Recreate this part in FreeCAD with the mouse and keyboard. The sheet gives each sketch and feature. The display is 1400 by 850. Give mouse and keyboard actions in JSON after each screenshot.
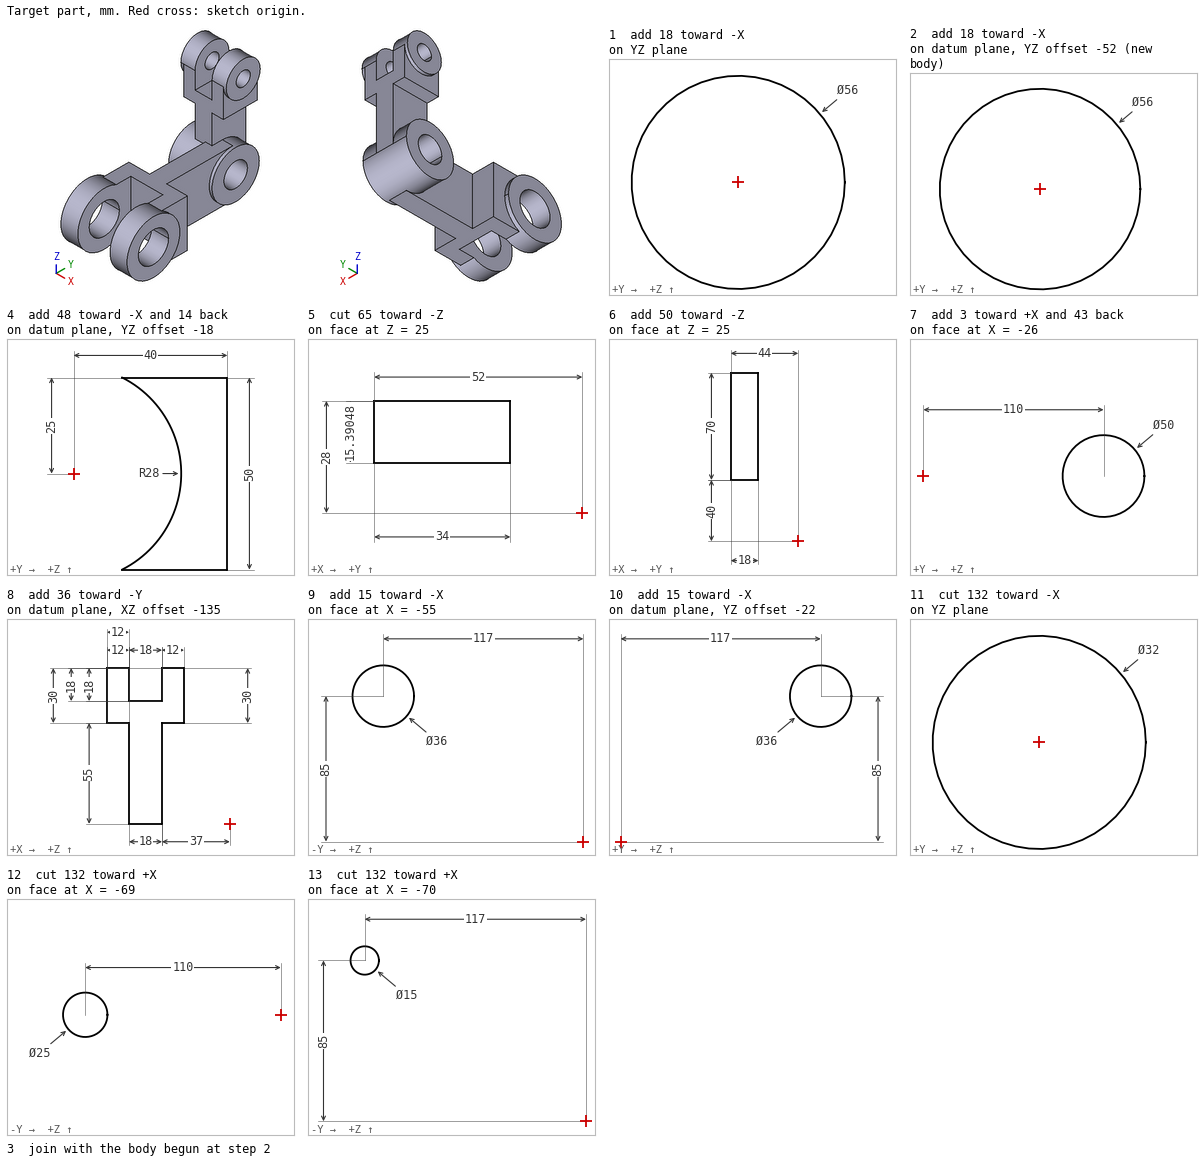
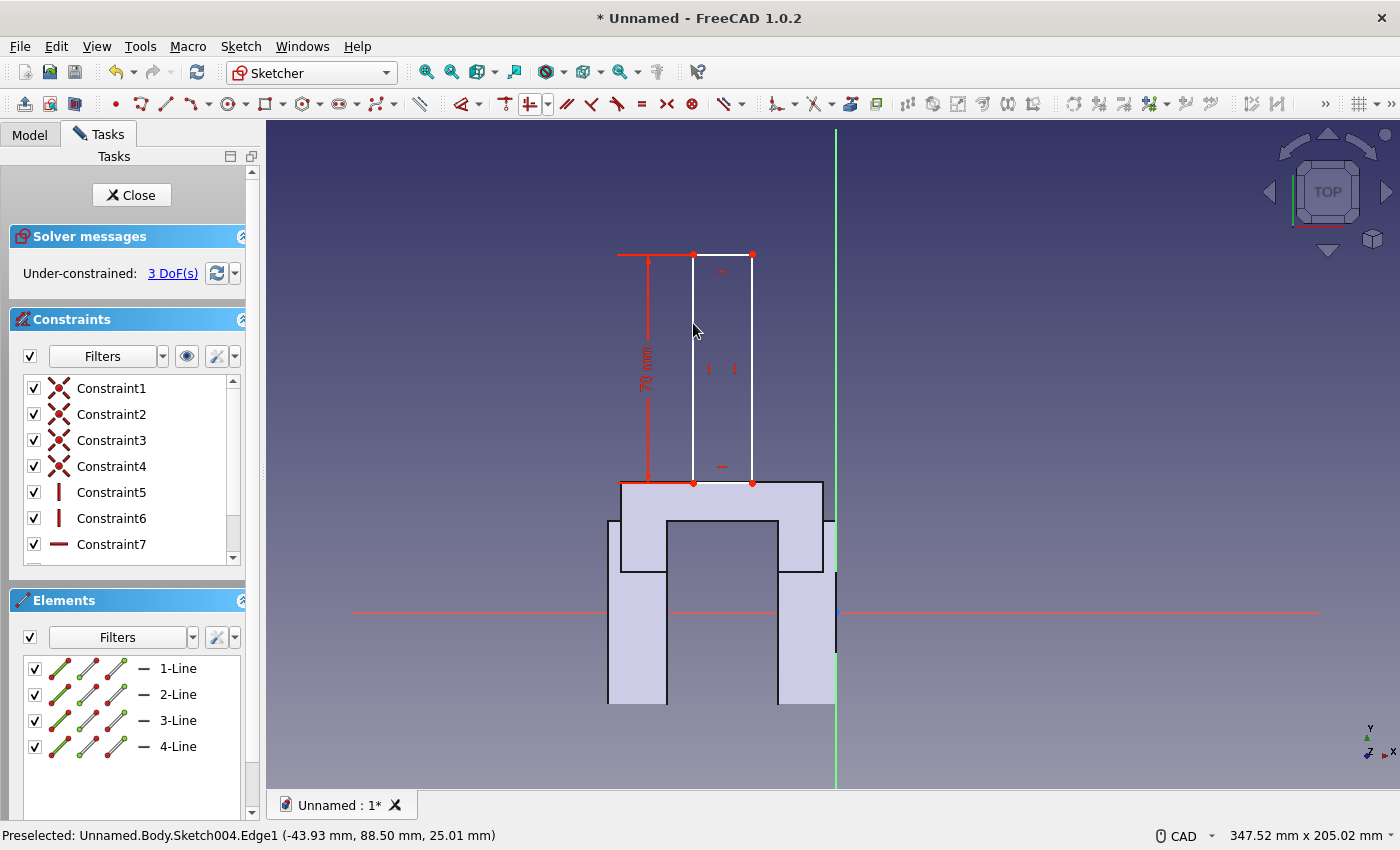
{"action": "left_click", "coordinate": [711, 483]}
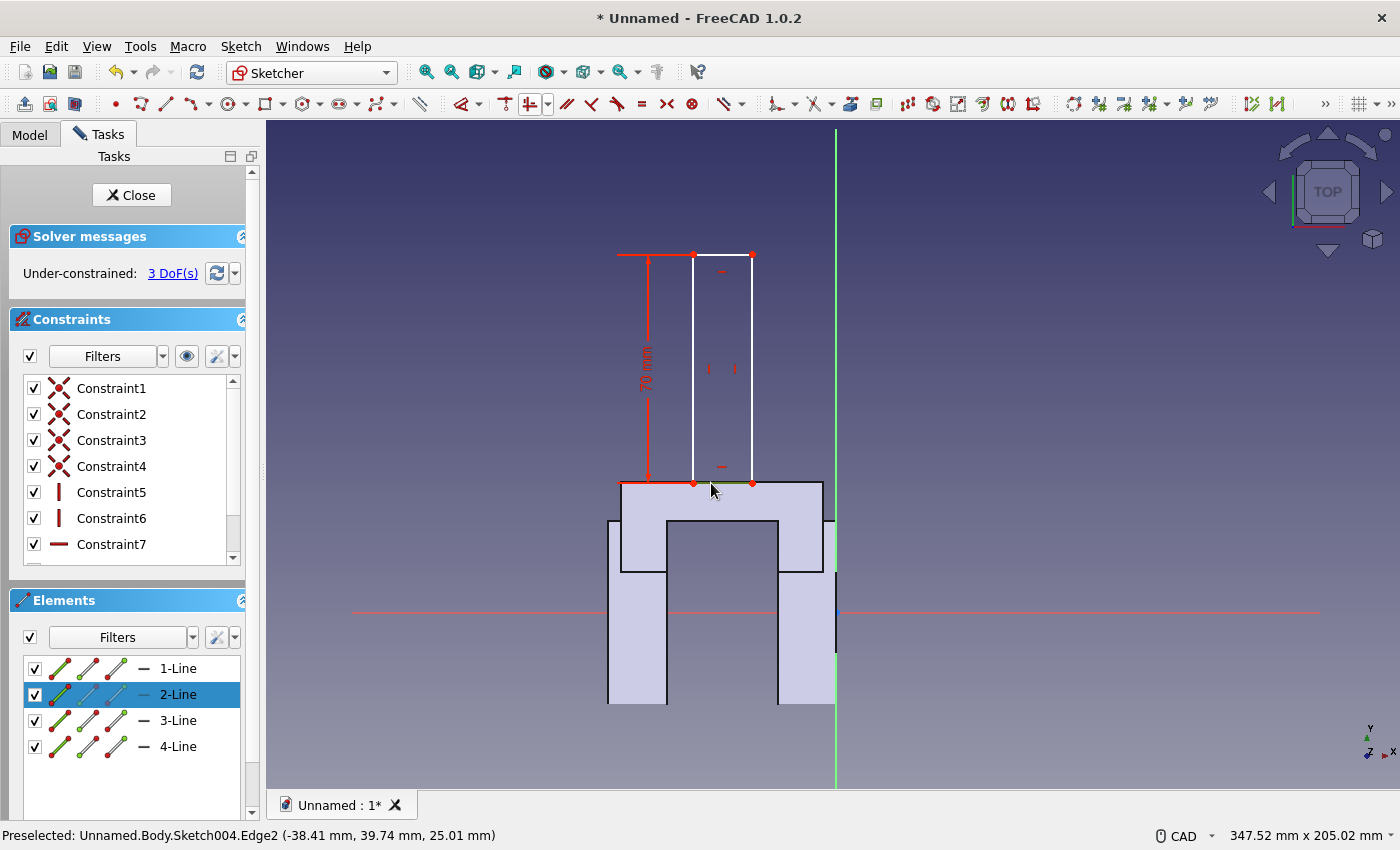
{"action": "key", "text": "l"}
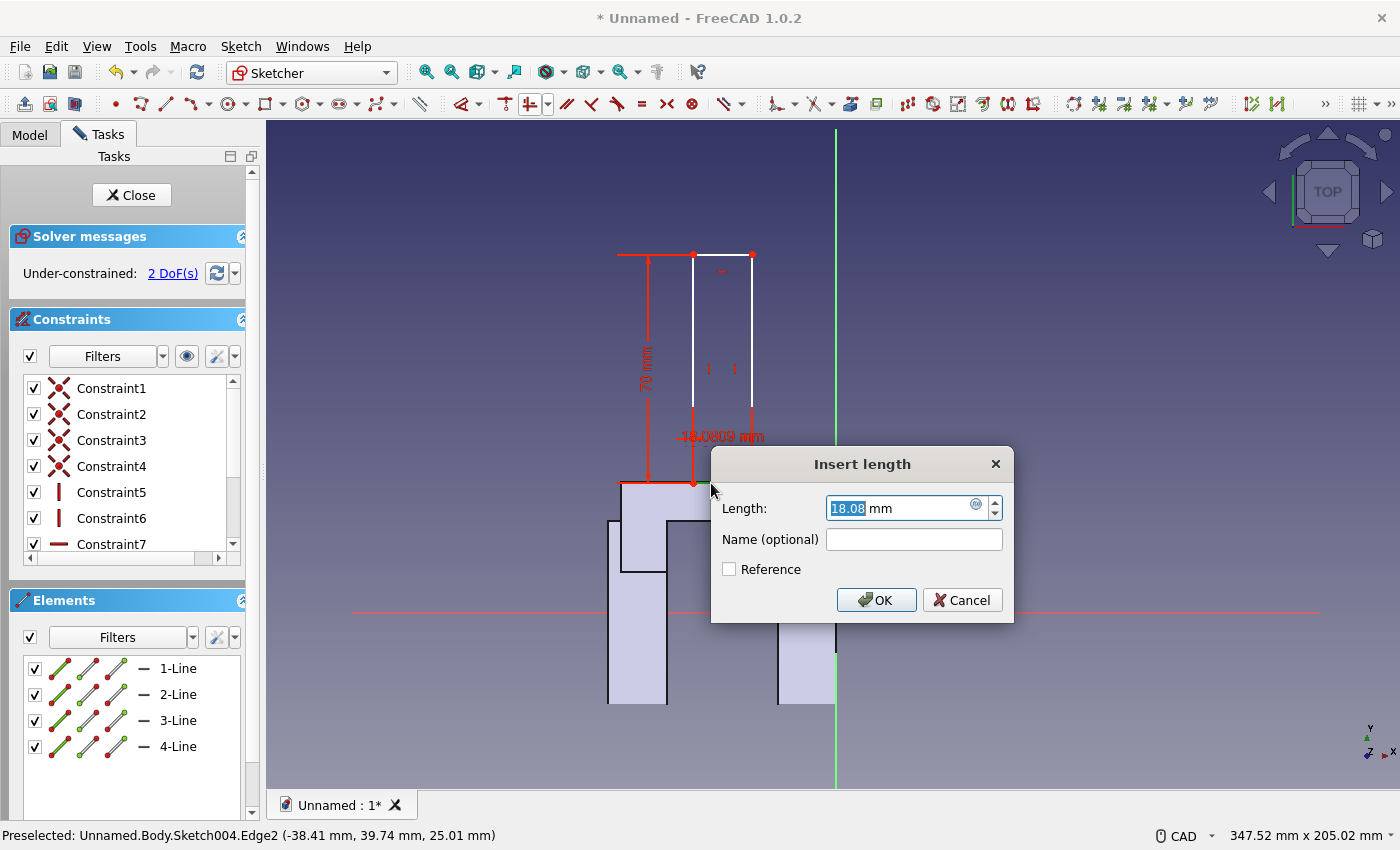
{"action": "type", "text": "18"}
{"action": "key", "text": "Return"}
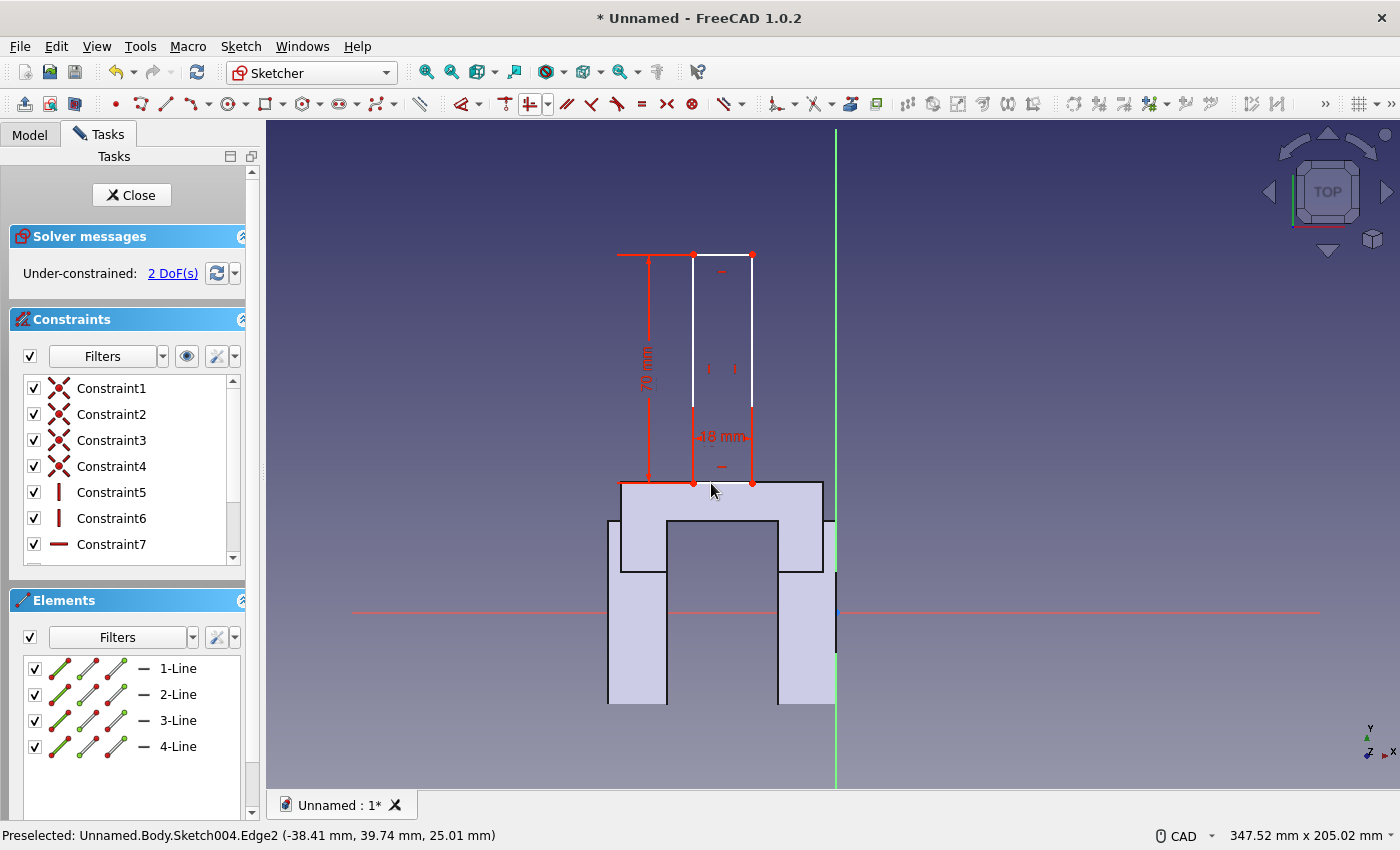
{"action": "left_click", "coordinate": [693, 255]}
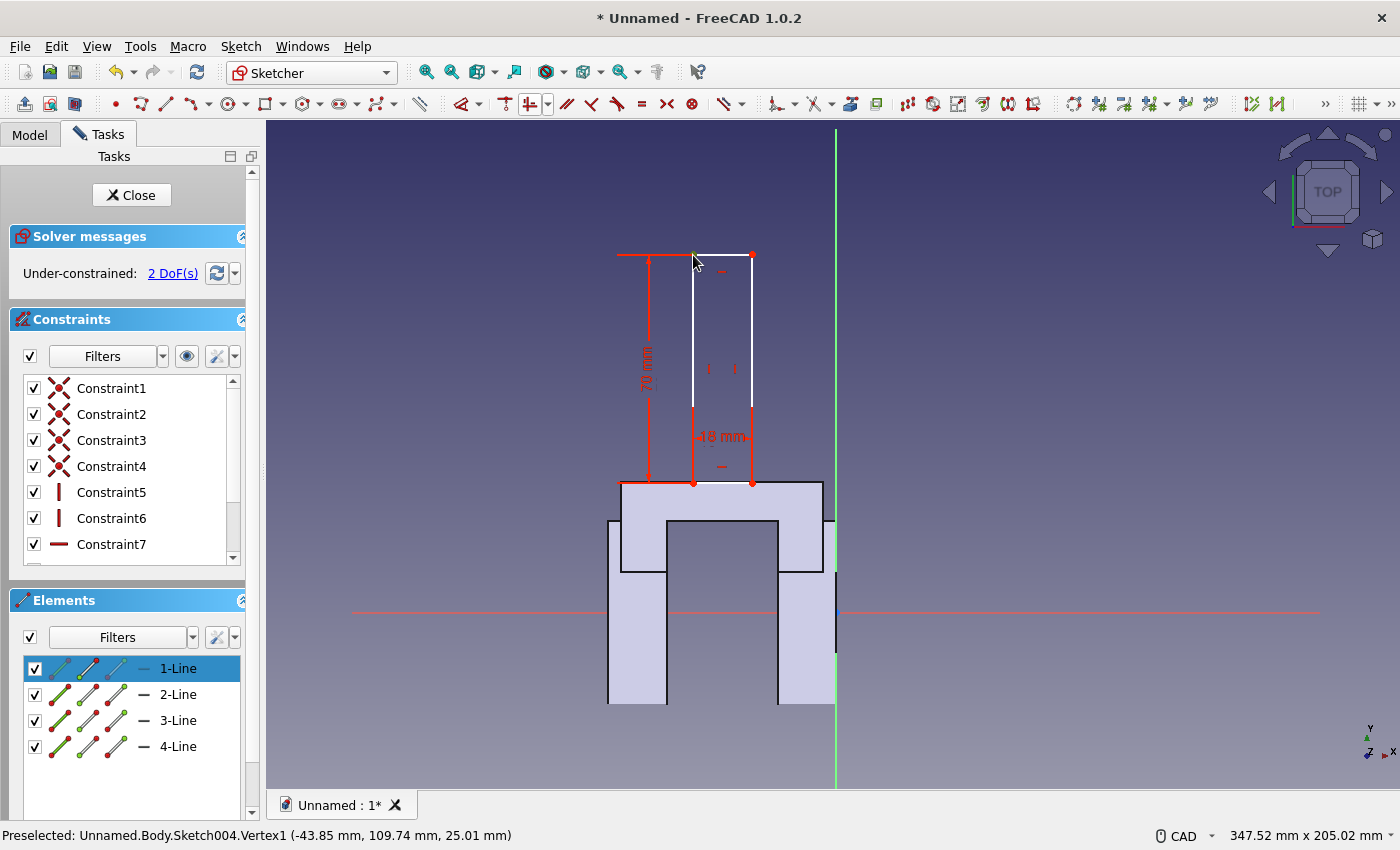
{"action": "key", "text": "l"}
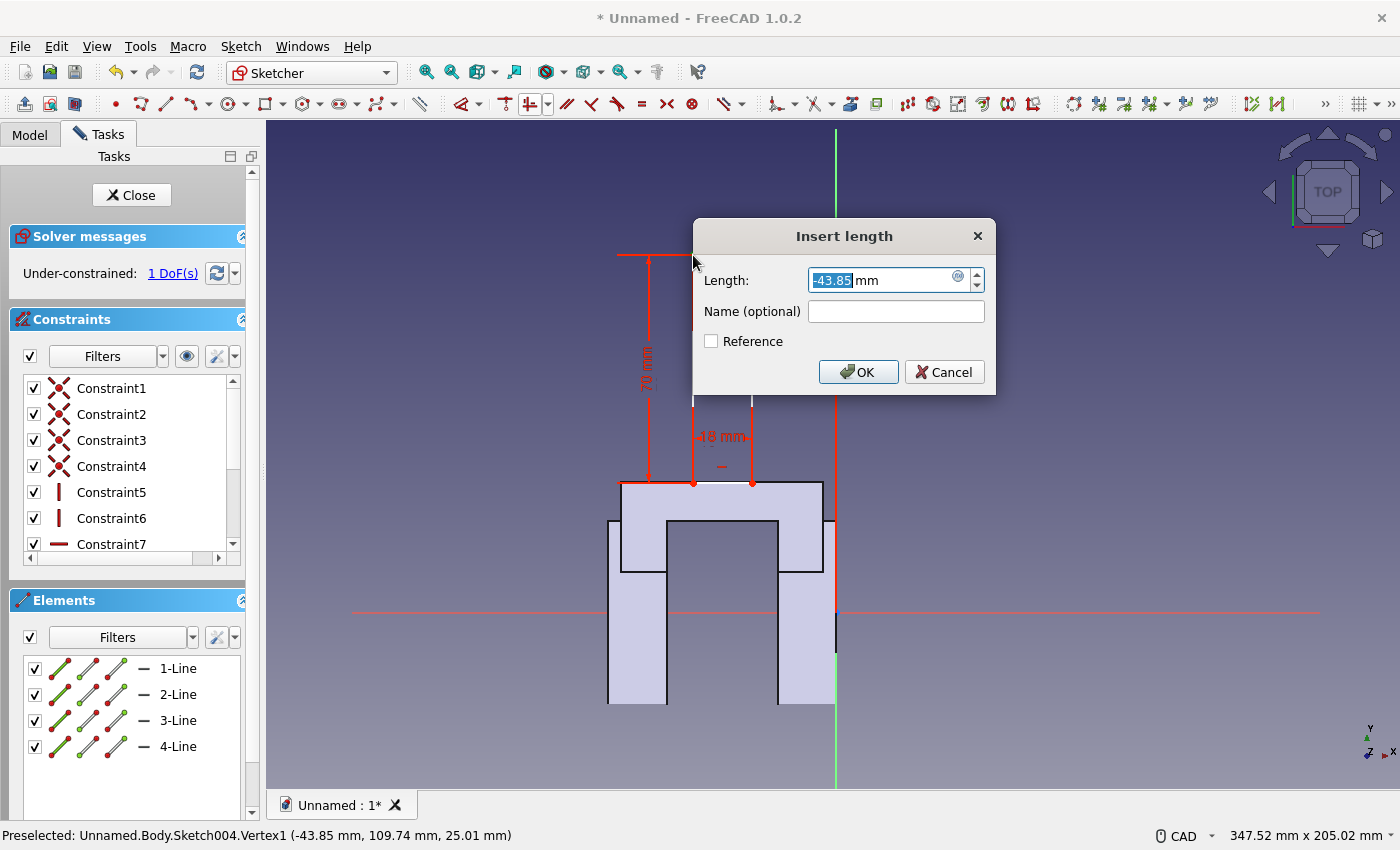
{"action": "type", "text": "-44"}
{"action": "key", "text": "Return"}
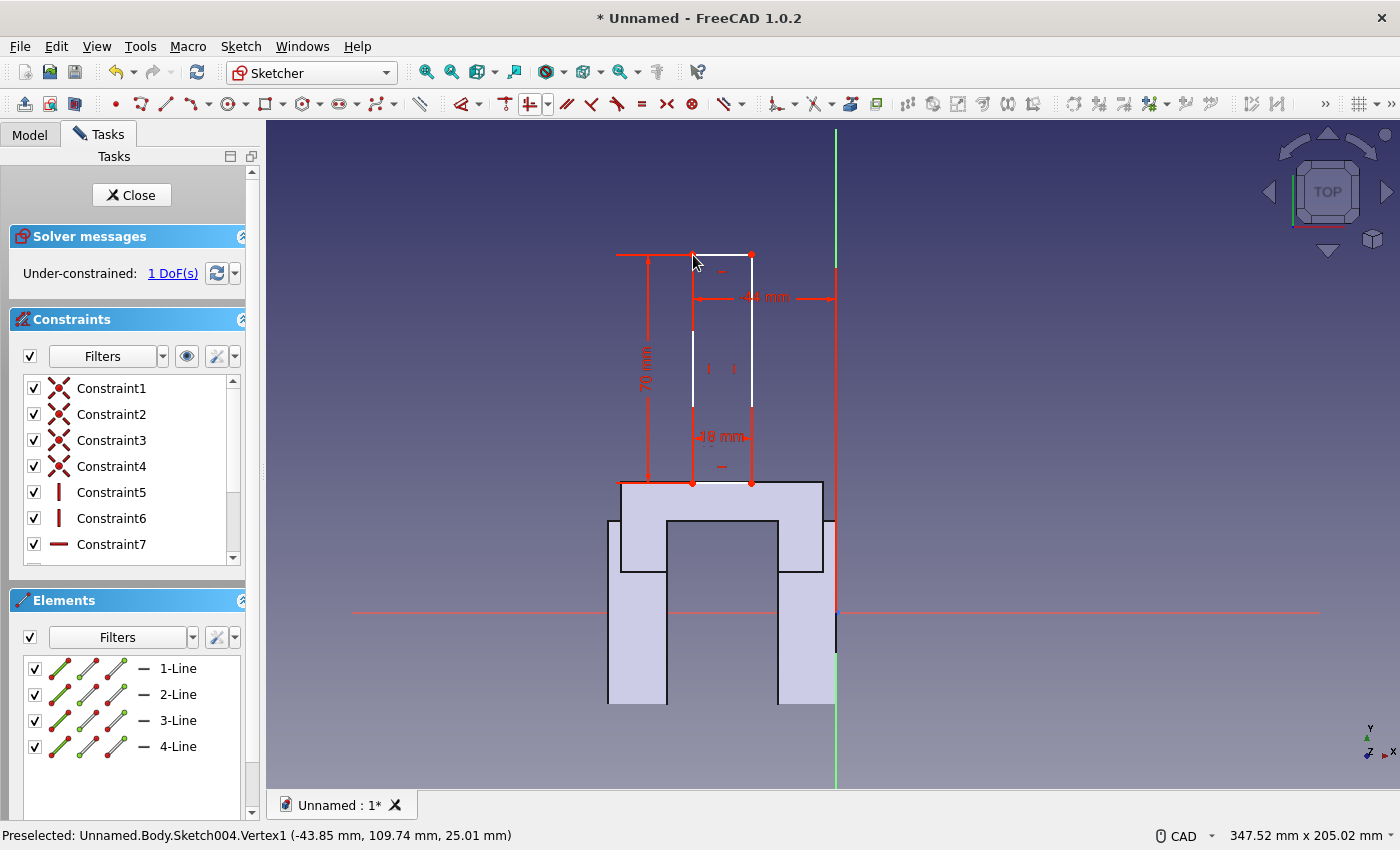
{"action": "left_click", "coordinate": [693, 483]}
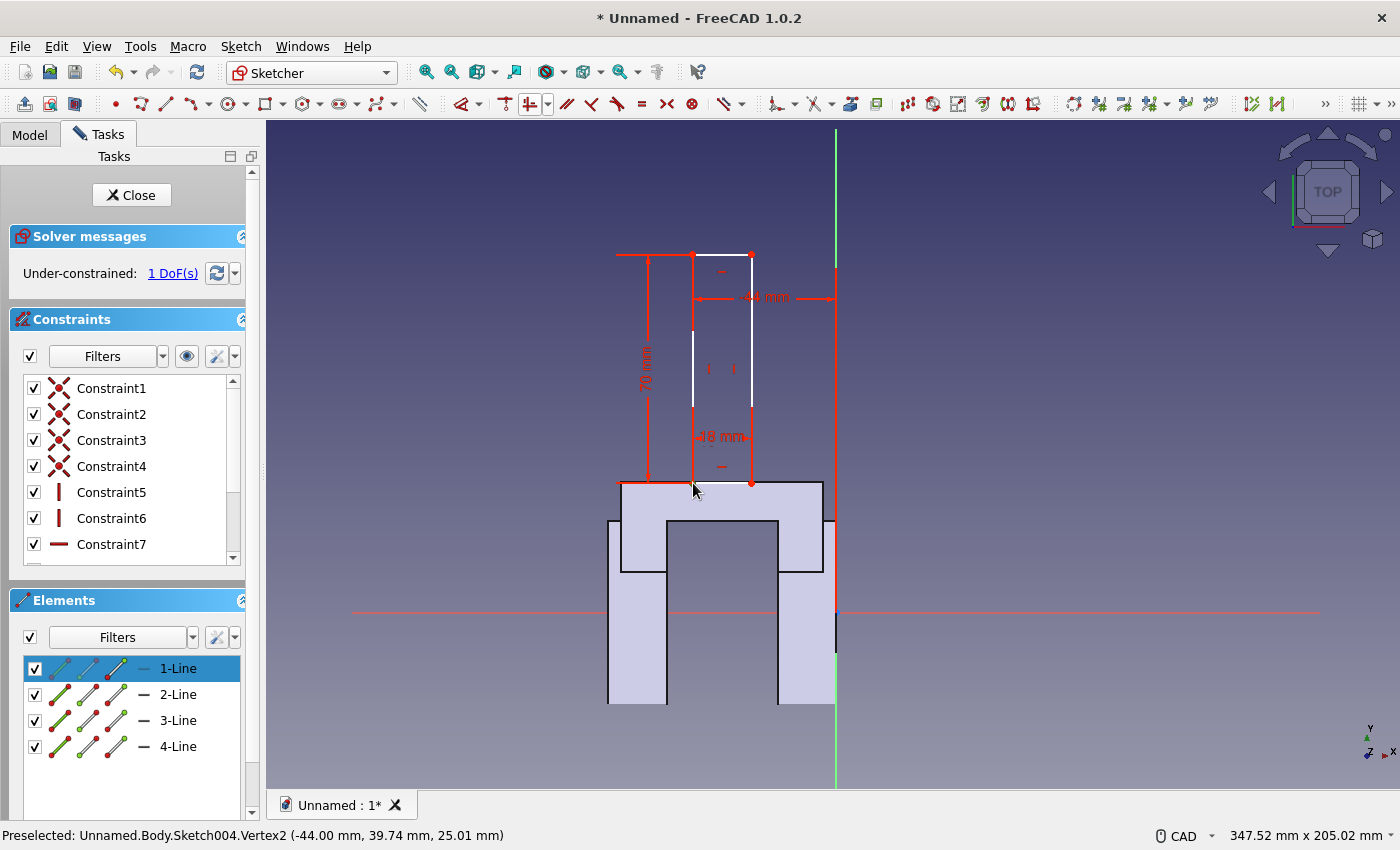
{"action": "key", "text": "i"}